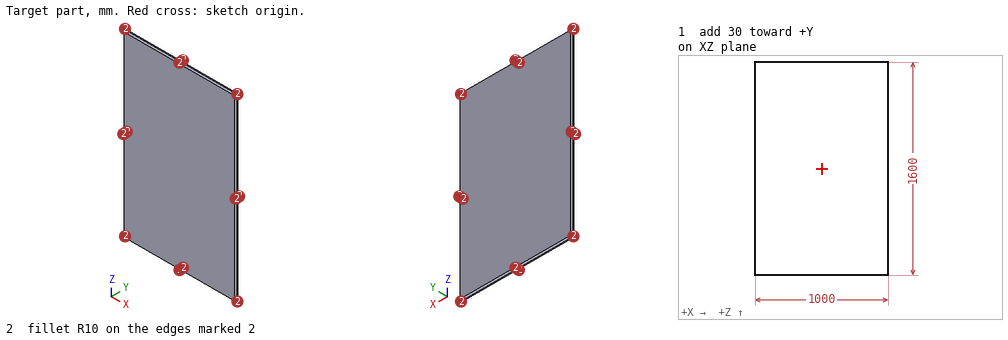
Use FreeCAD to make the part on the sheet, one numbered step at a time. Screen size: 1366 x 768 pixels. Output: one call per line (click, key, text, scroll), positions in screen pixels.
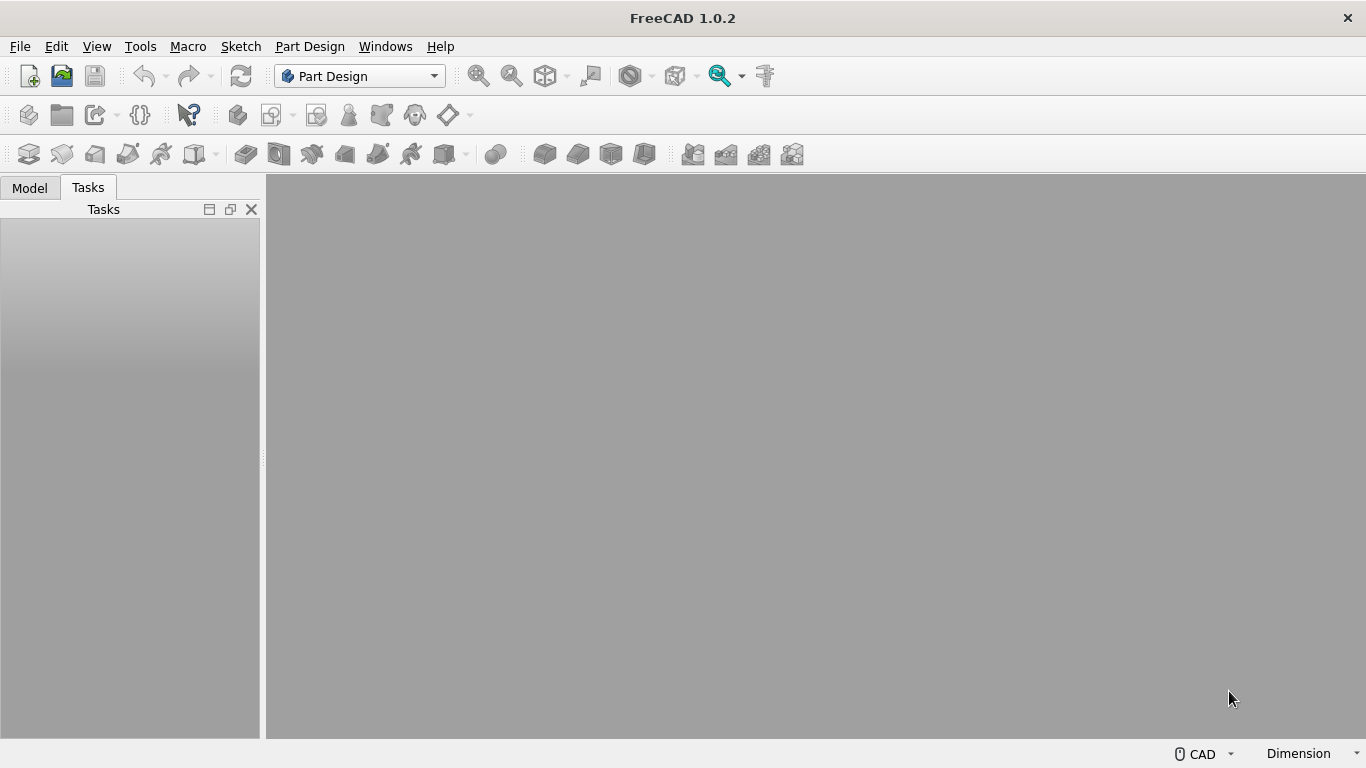
click(29, 76)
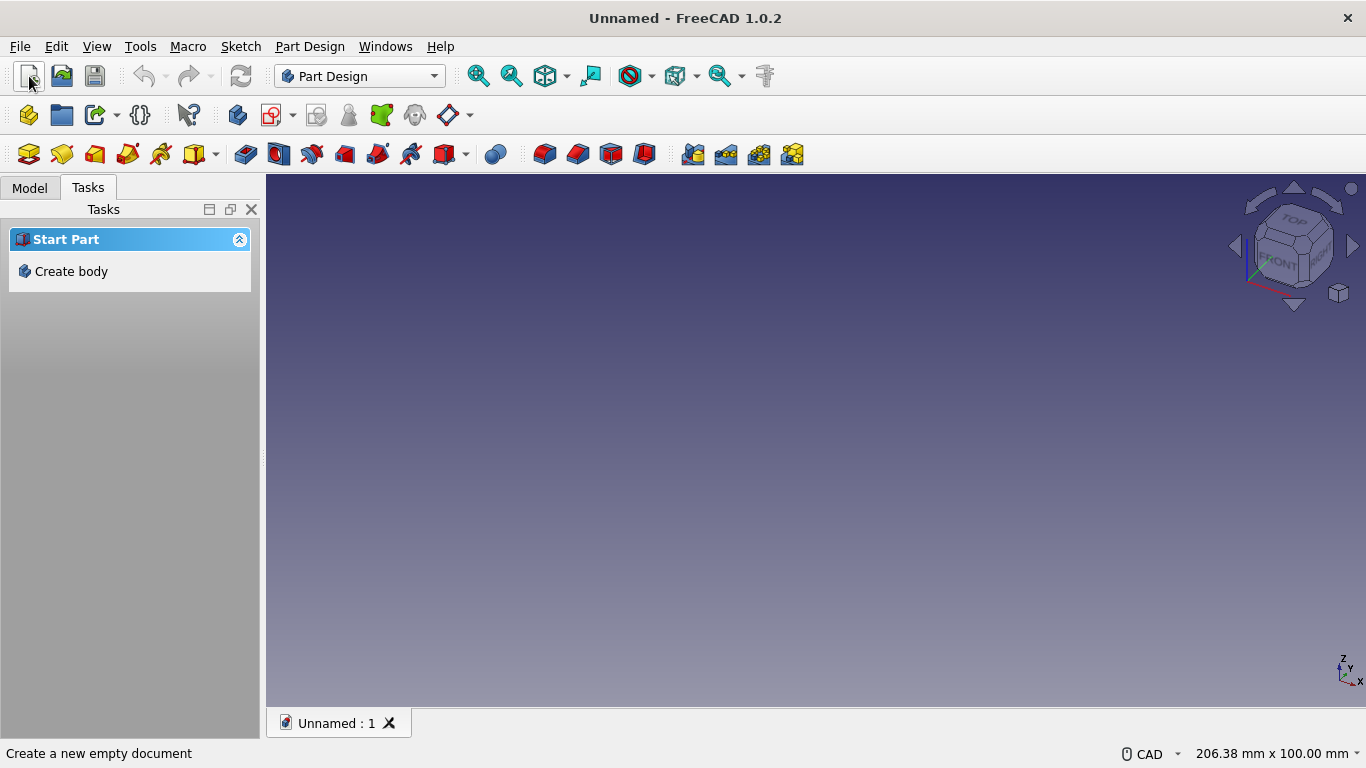
click(270, 116)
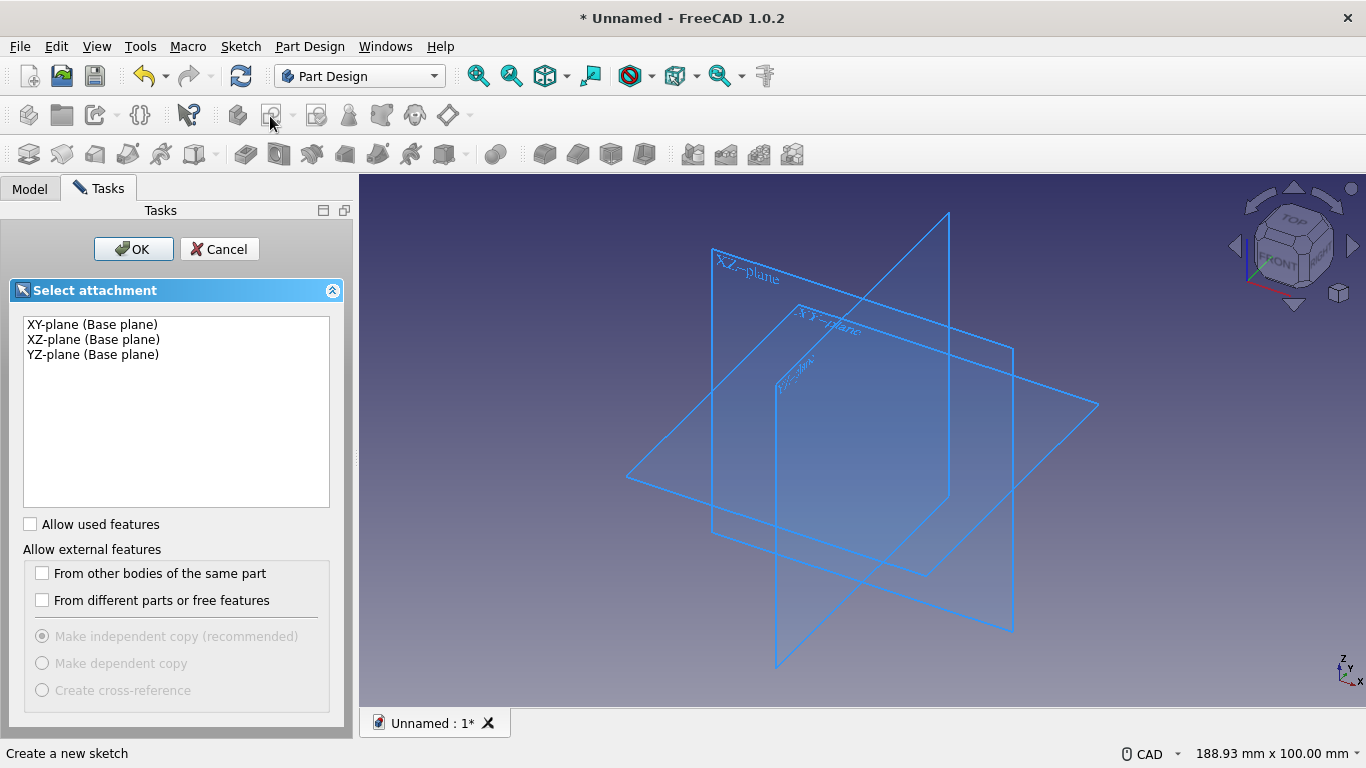
click(84, 340)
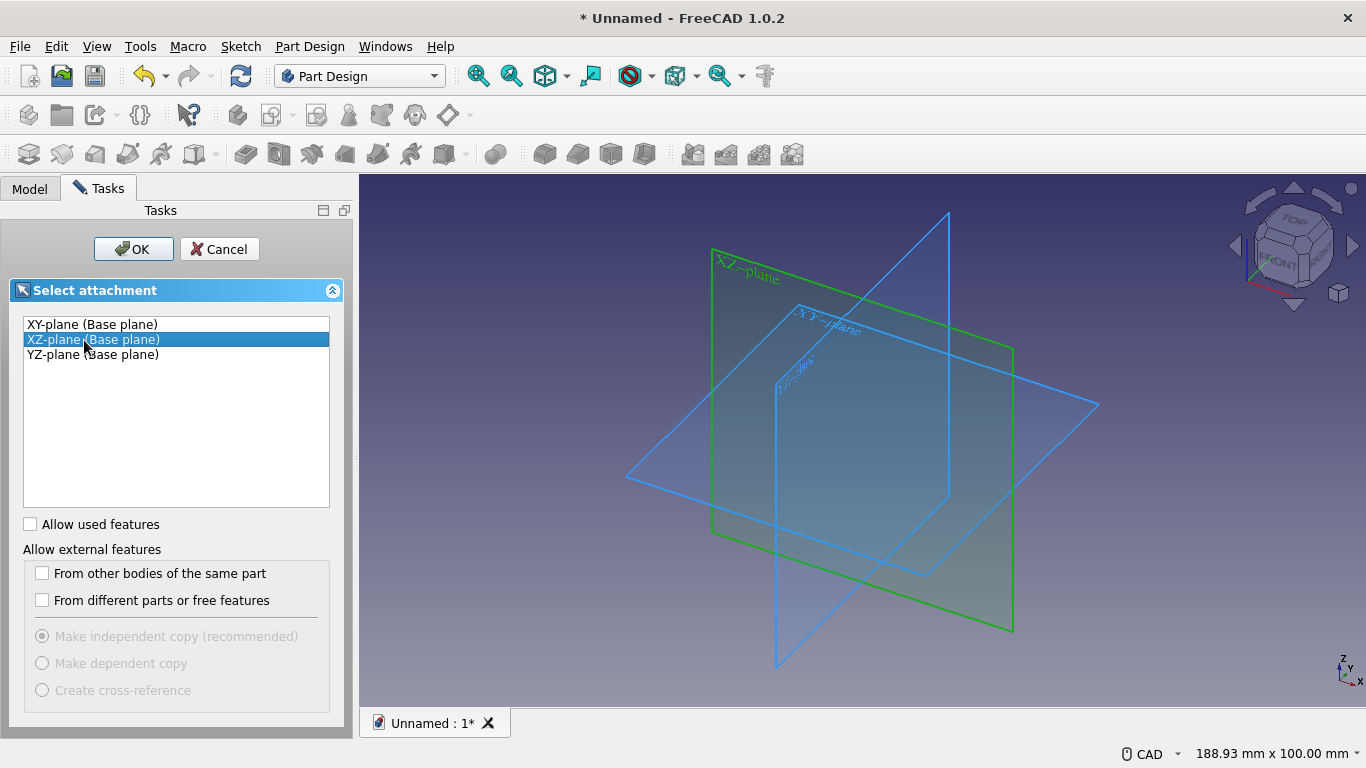
click(134, 249)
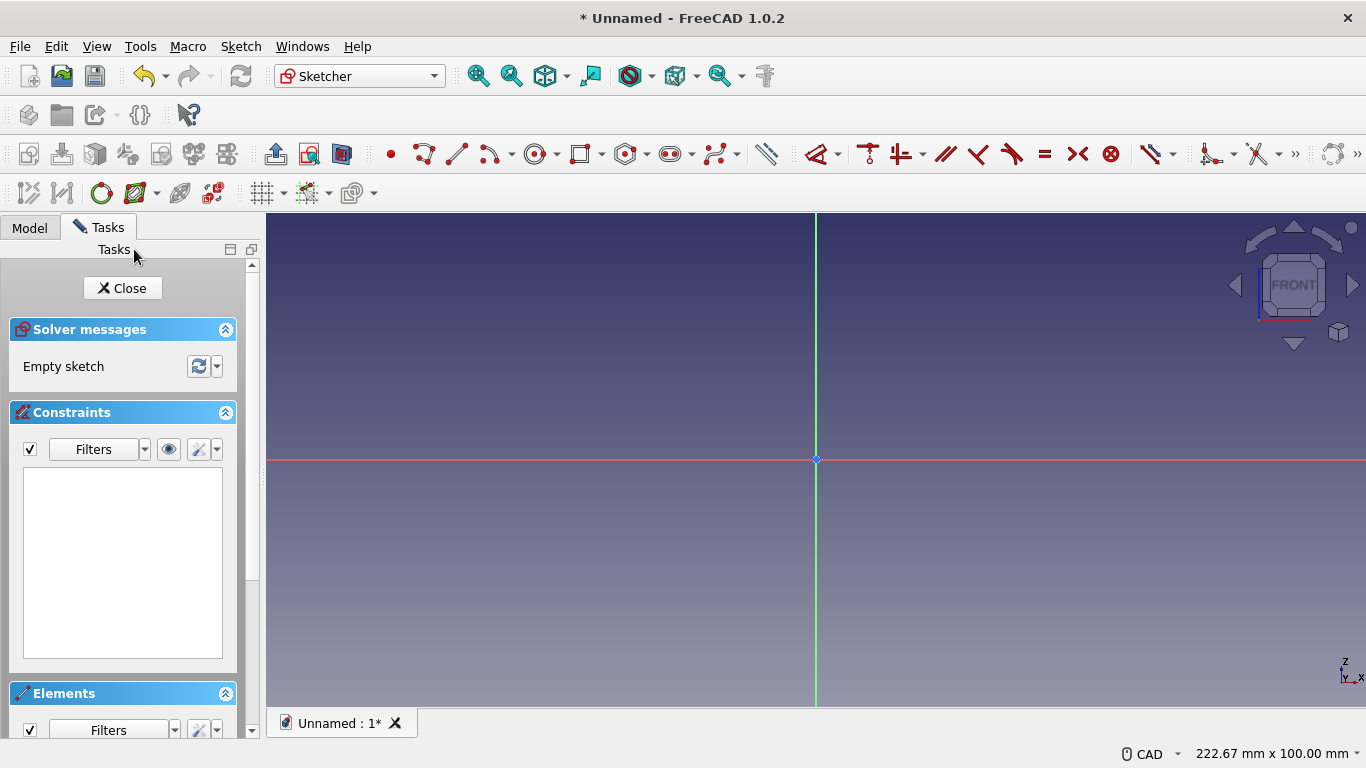
scroll(745, 460, down, 16)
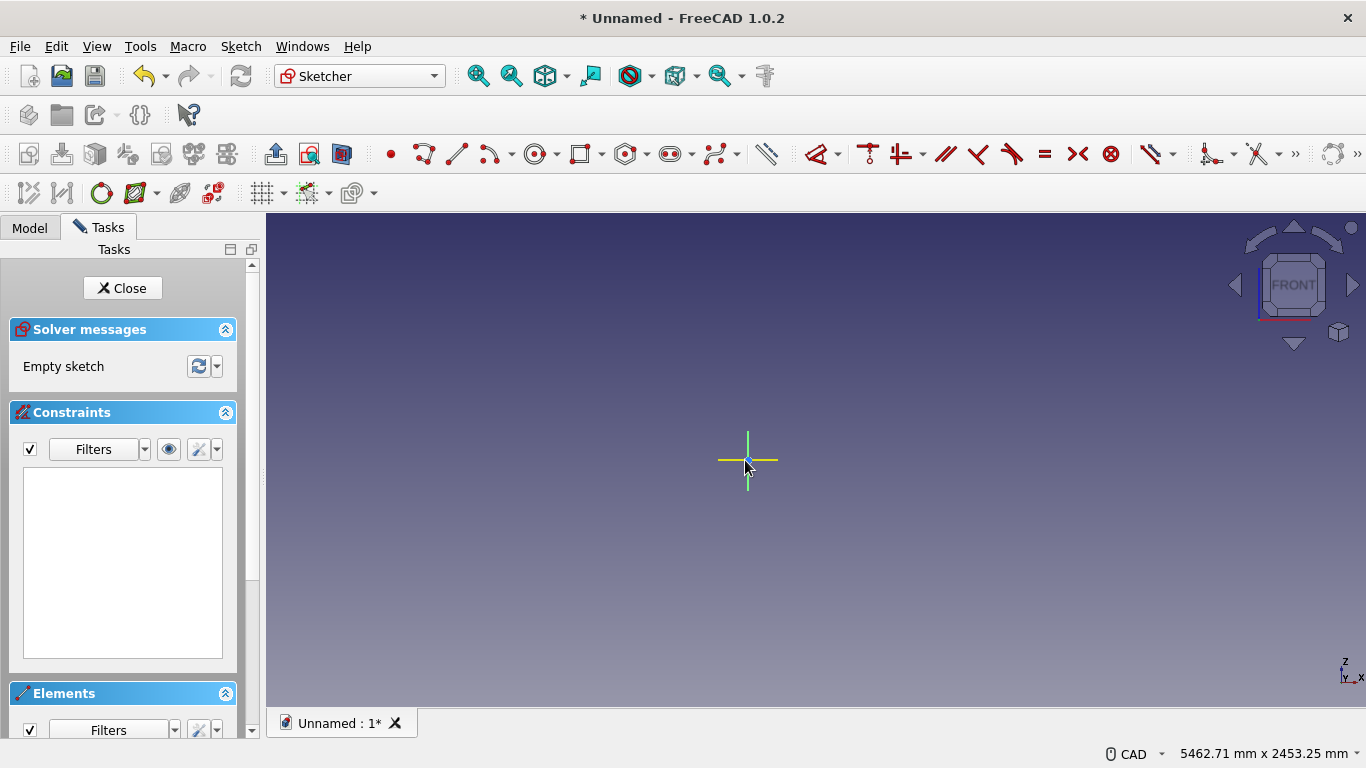
key(g)
key(v)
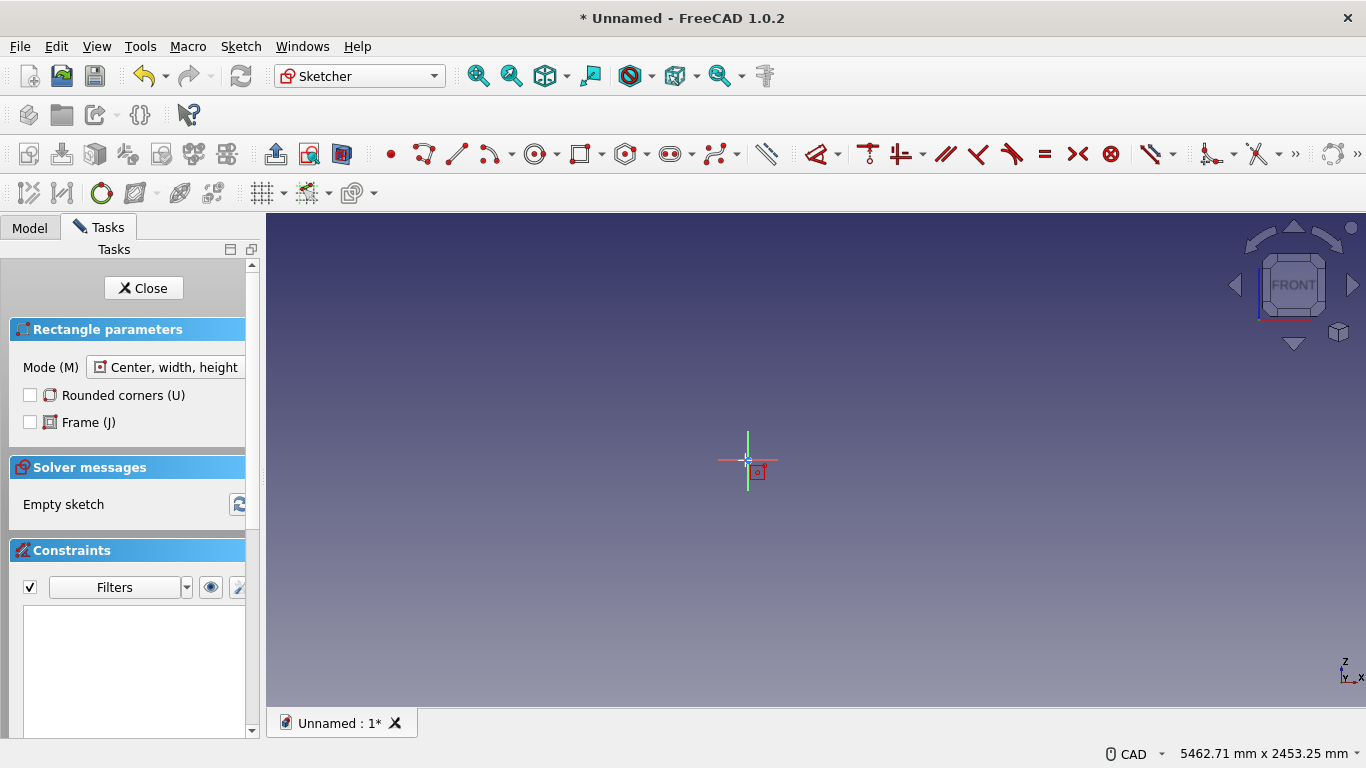
click(748, 460)
move(849, 299)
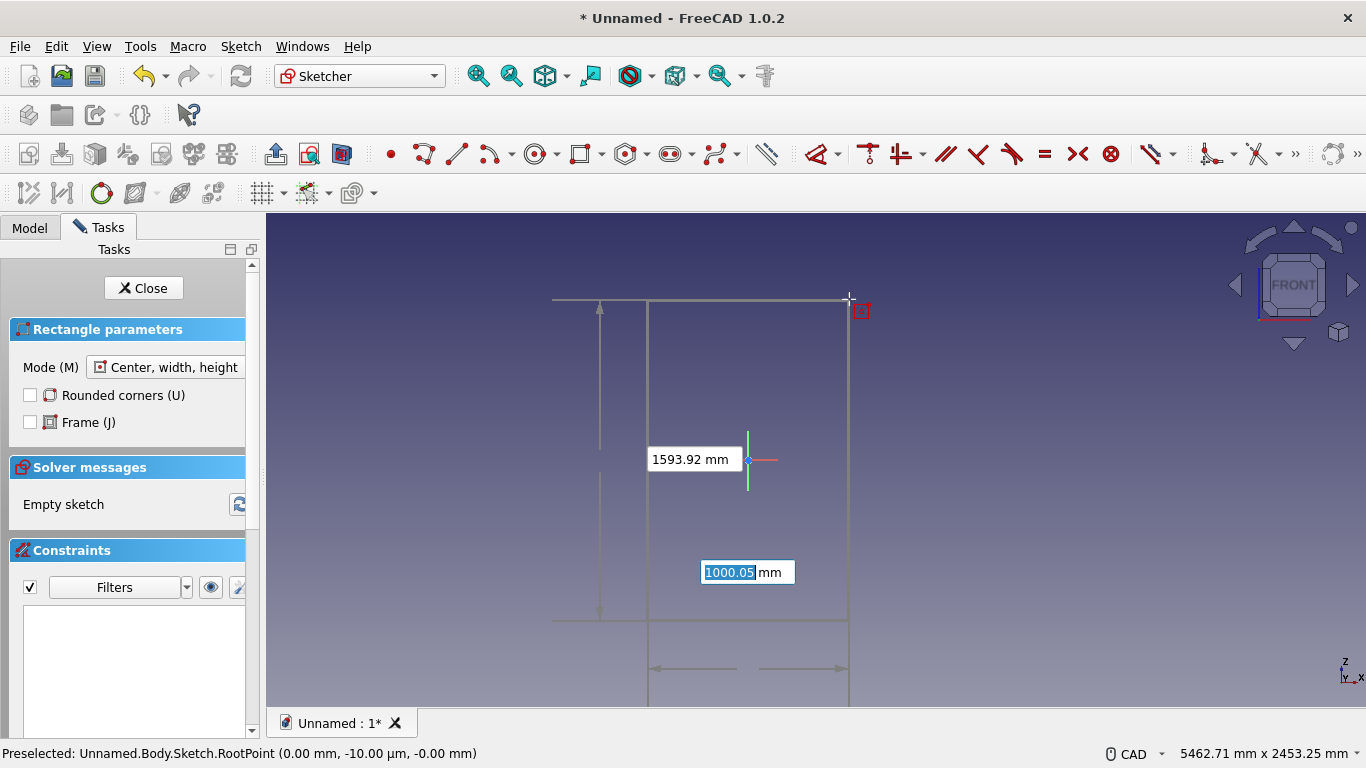
text(1000)
key(Tab)
text(1600)
key(Return)
key(Escape)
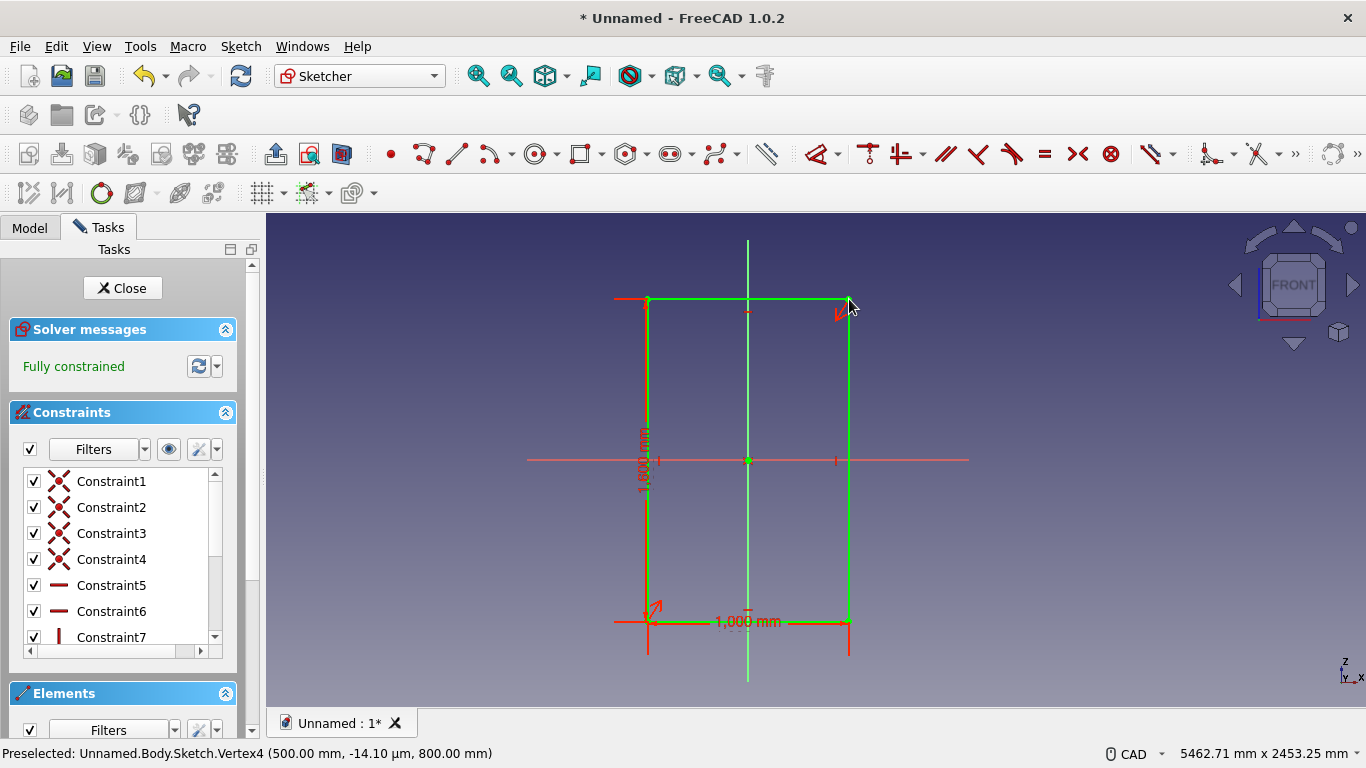
click(123, 288)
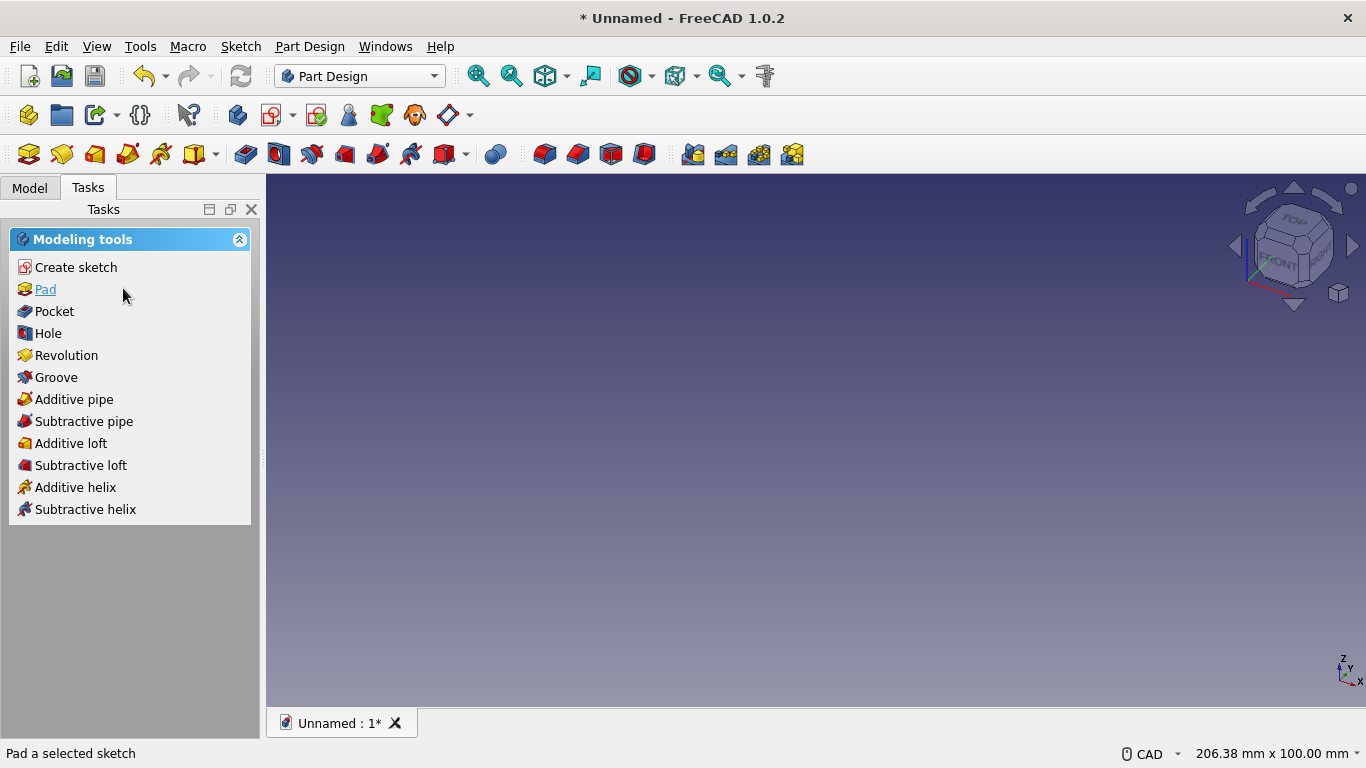
click(29, 154)